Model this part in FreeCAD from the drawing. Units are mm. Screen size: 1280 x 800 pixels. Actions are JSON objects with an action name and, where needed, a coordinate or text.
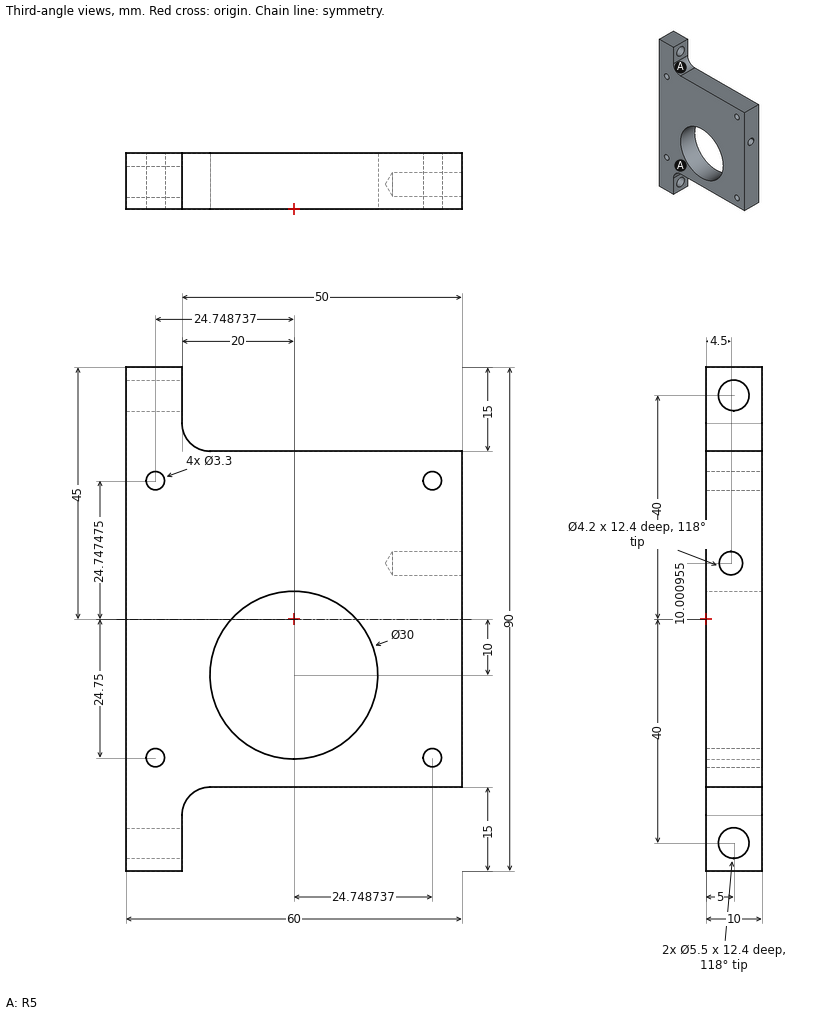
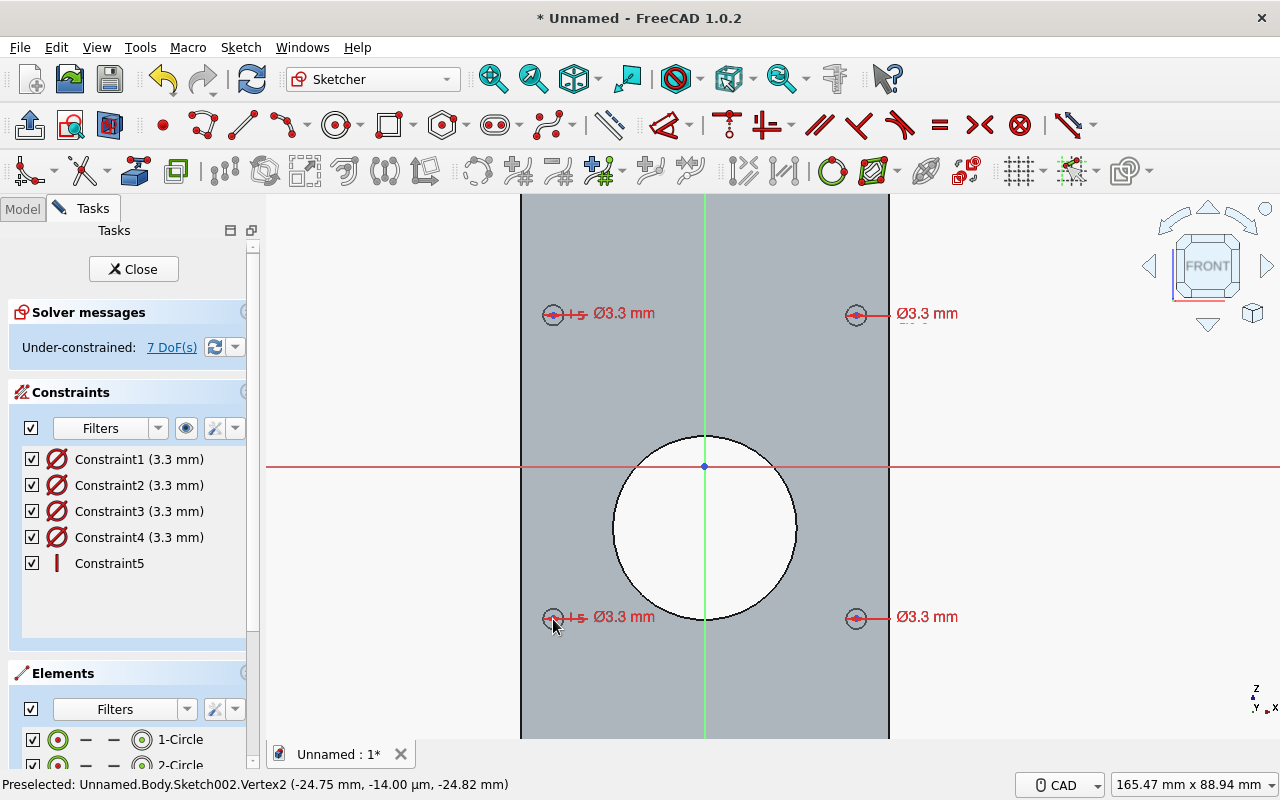
{"action": "left_click", "coordinate": [553, 619]}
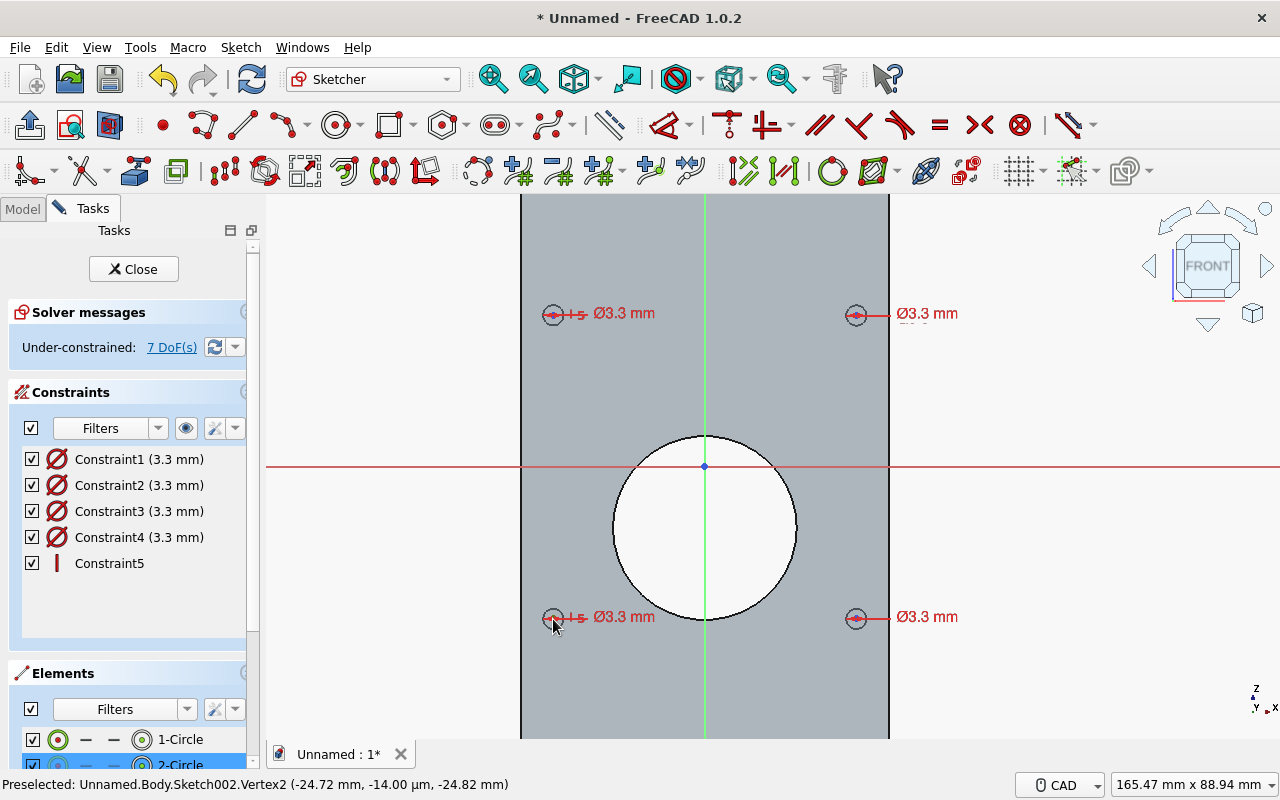
{"action": "left_click", "coordinate": [856, 619]}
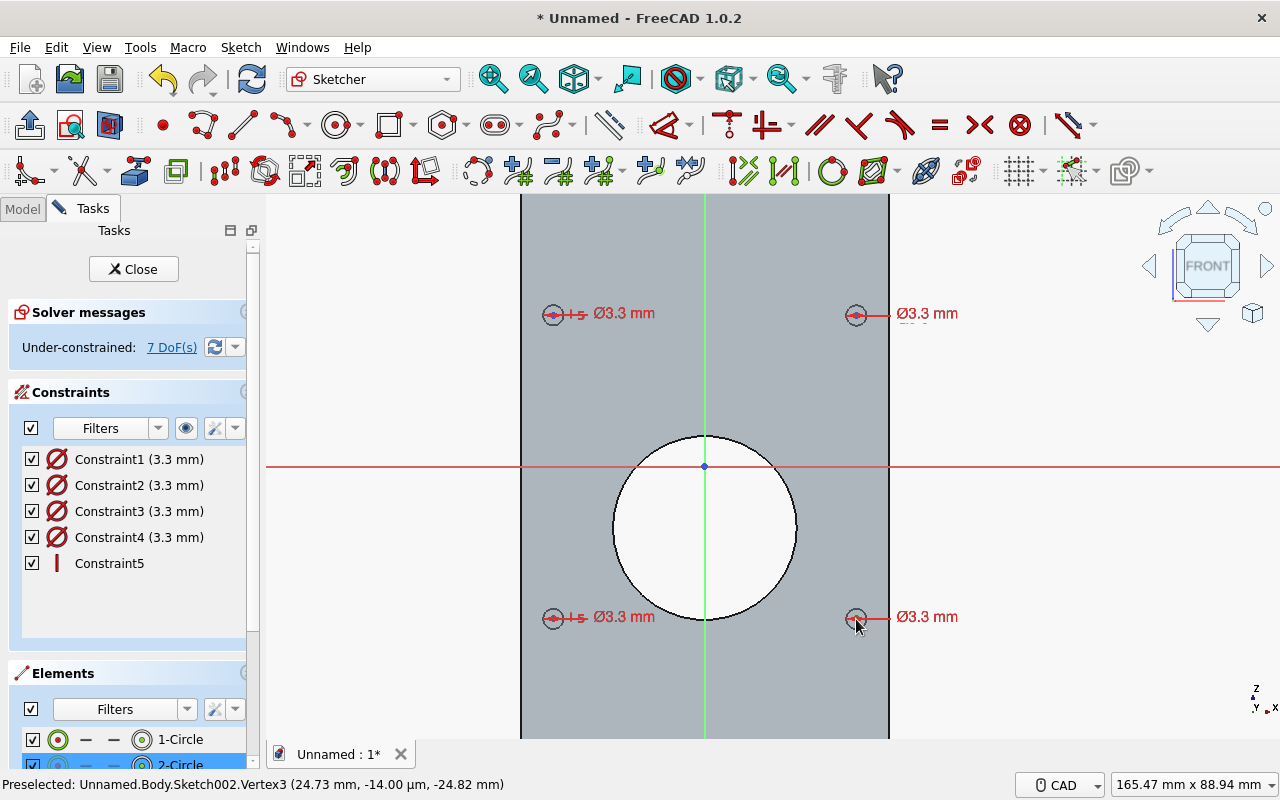
{"action": "key", "text": "h"}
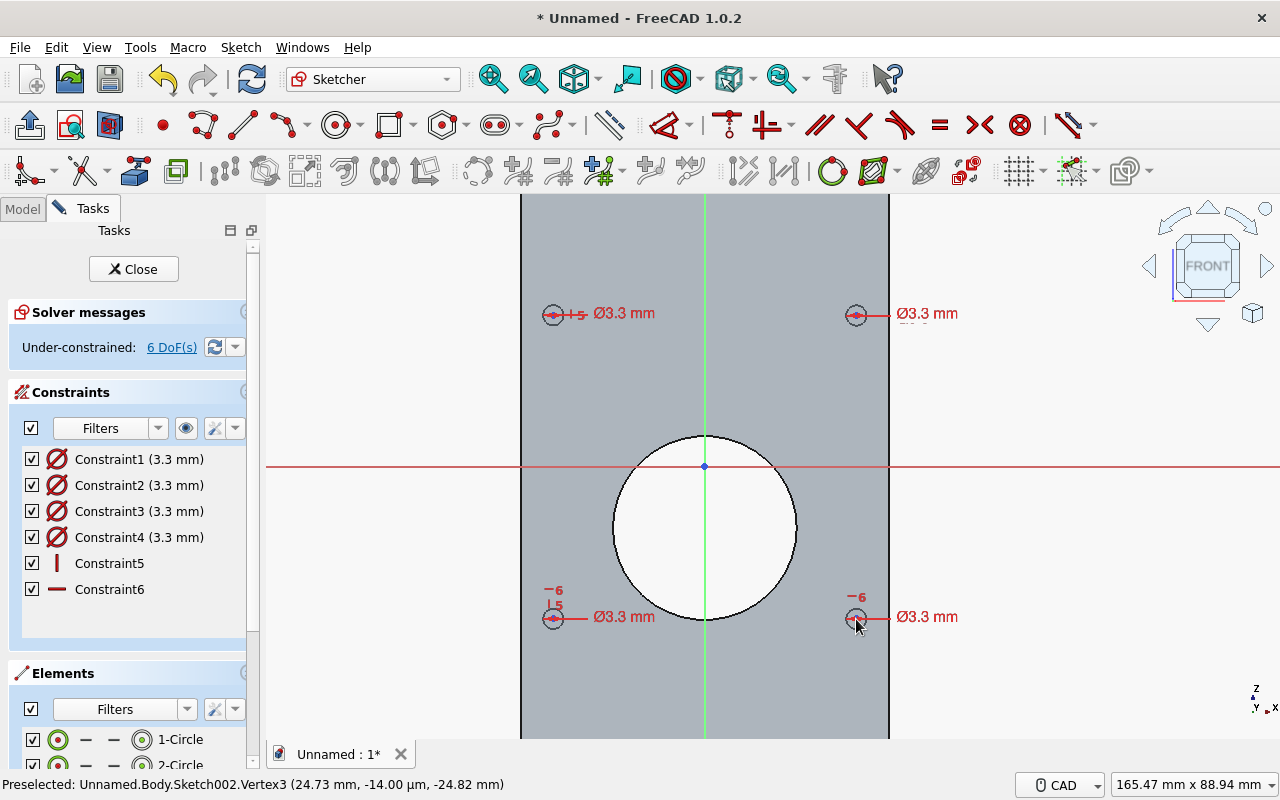
{"action": "left_click", "coordinate": [856, 619]}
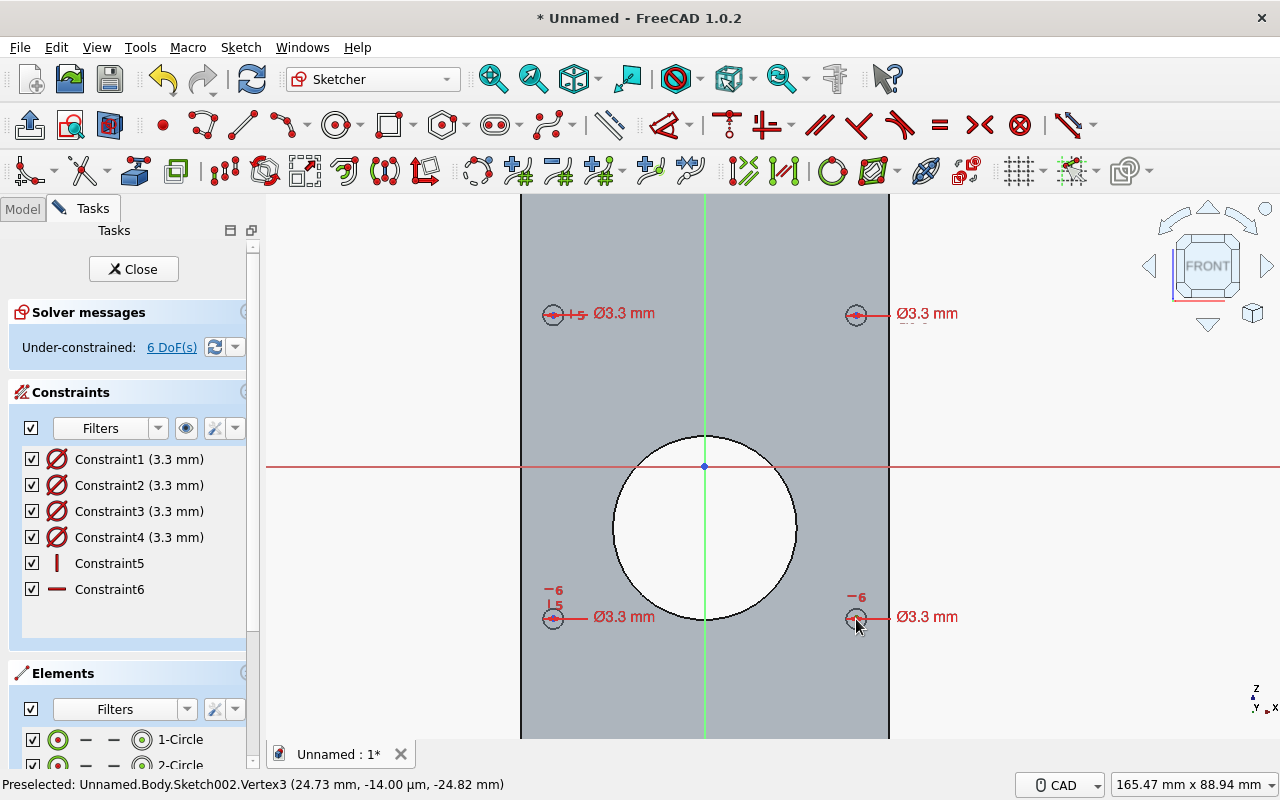
{"action": "left_click", "coordinate": [856, 316]}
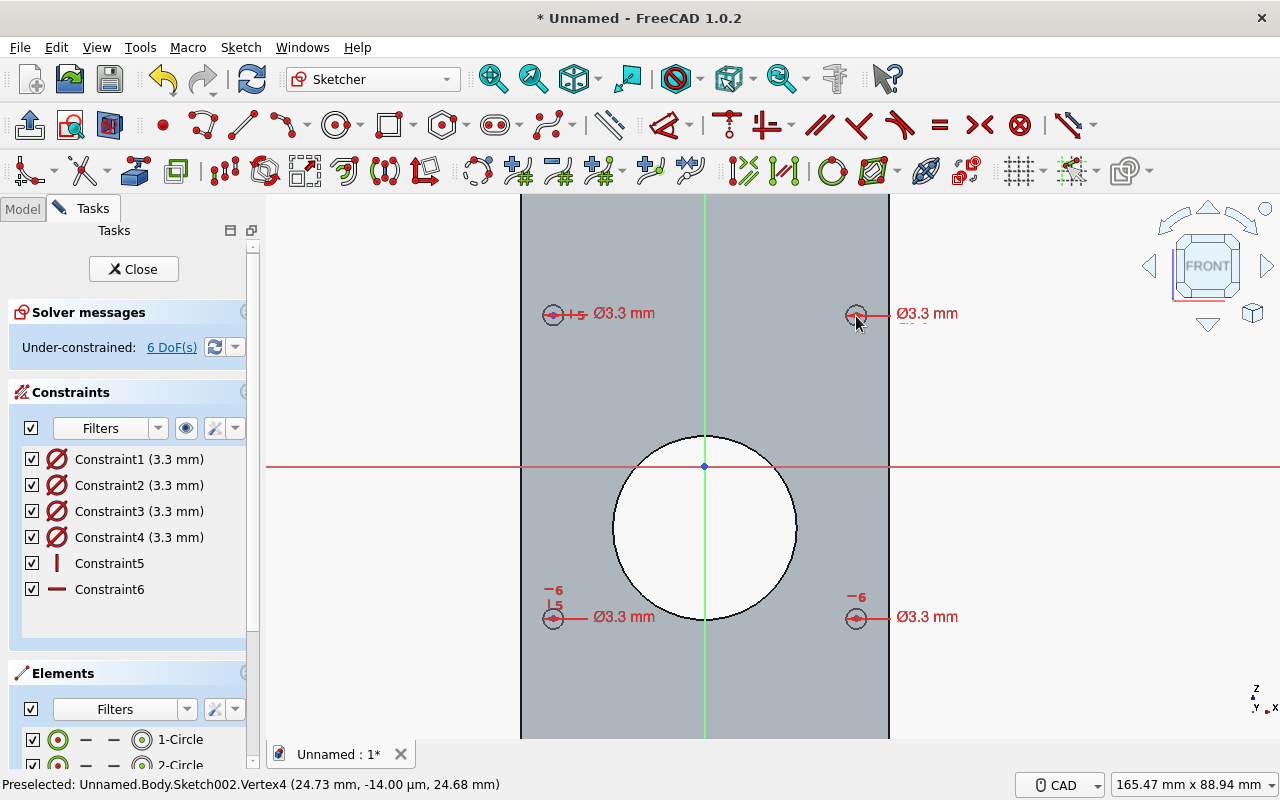
{"action": "key", "text": "v"}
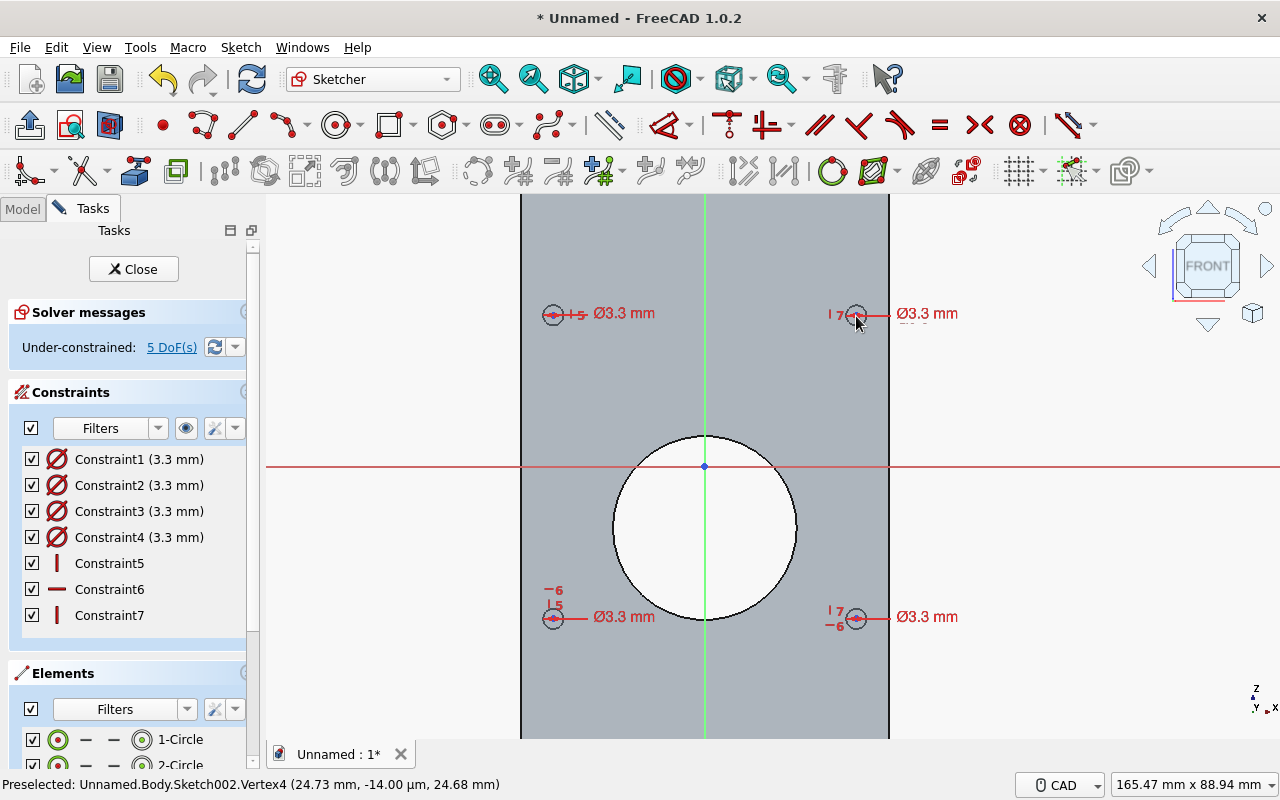
{"action": "left_click", "coordinate": [553, 315]}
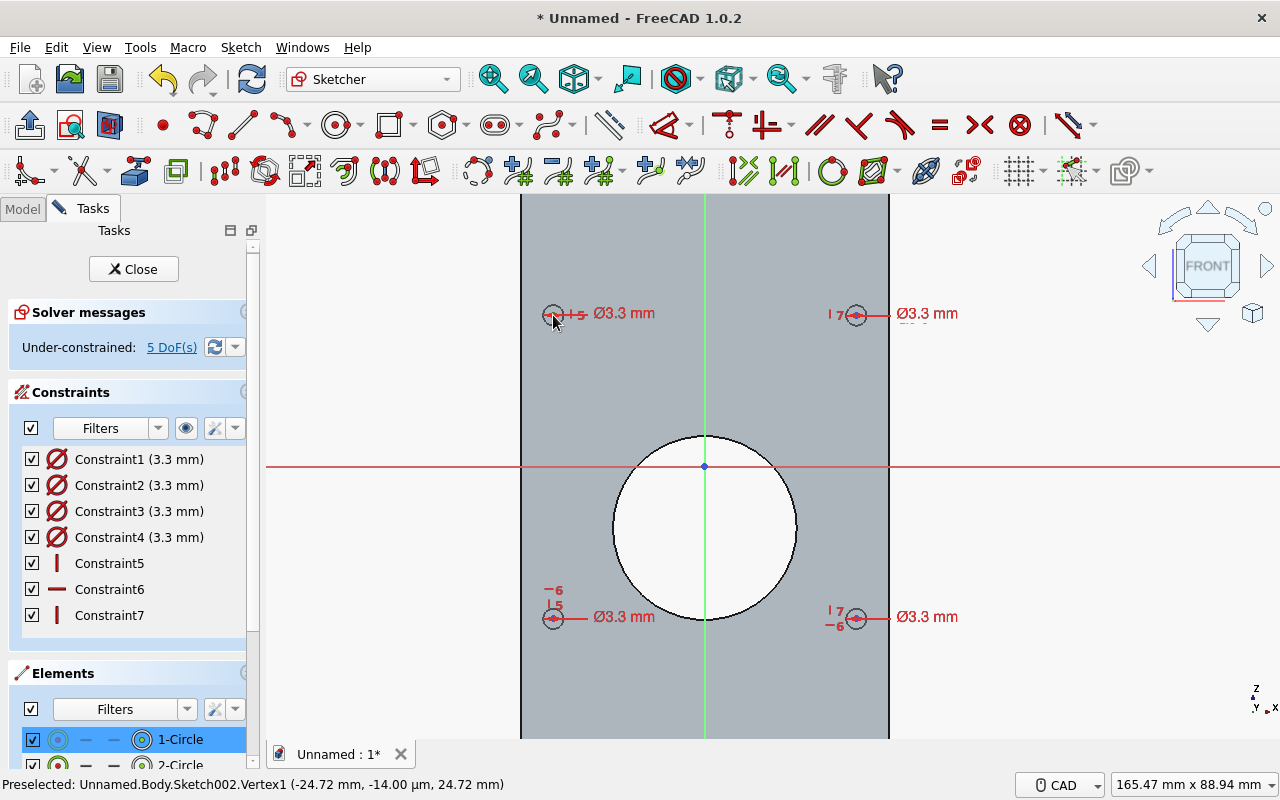
{"action": "left_click", "coordinate": [856, 316]}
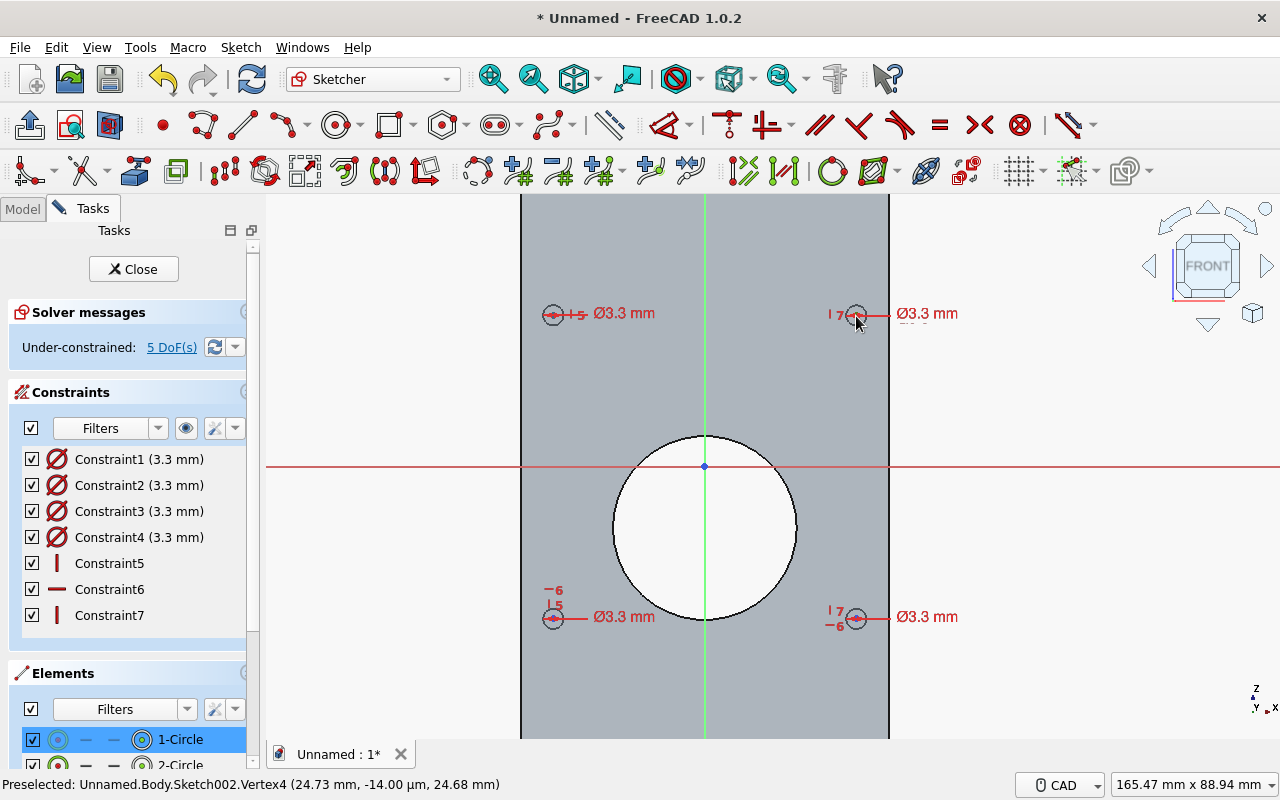
{"action": "key", "text": "h"}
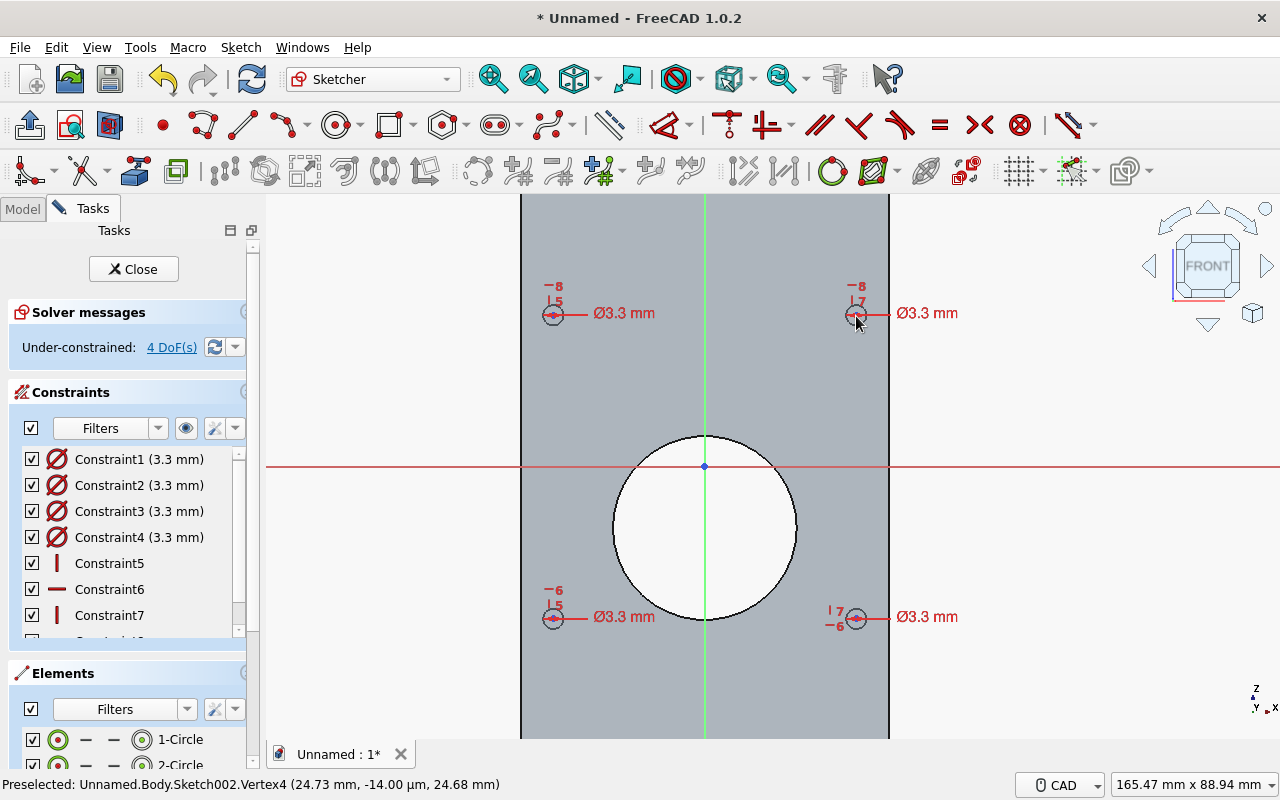
{"action": "left_click", "coordinate": [664, 126]}